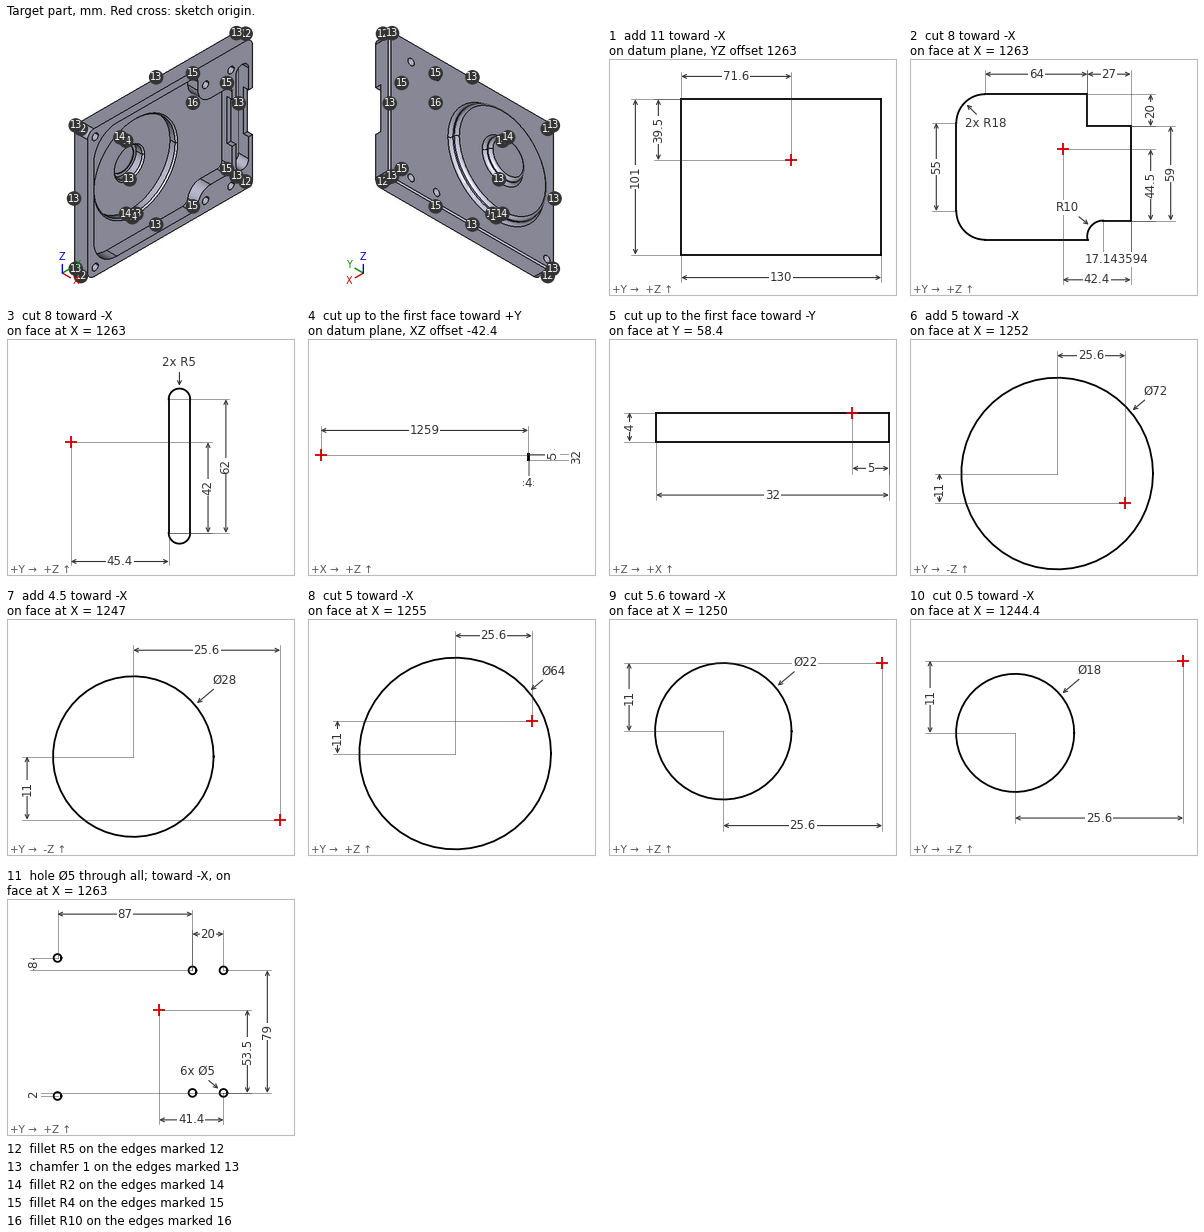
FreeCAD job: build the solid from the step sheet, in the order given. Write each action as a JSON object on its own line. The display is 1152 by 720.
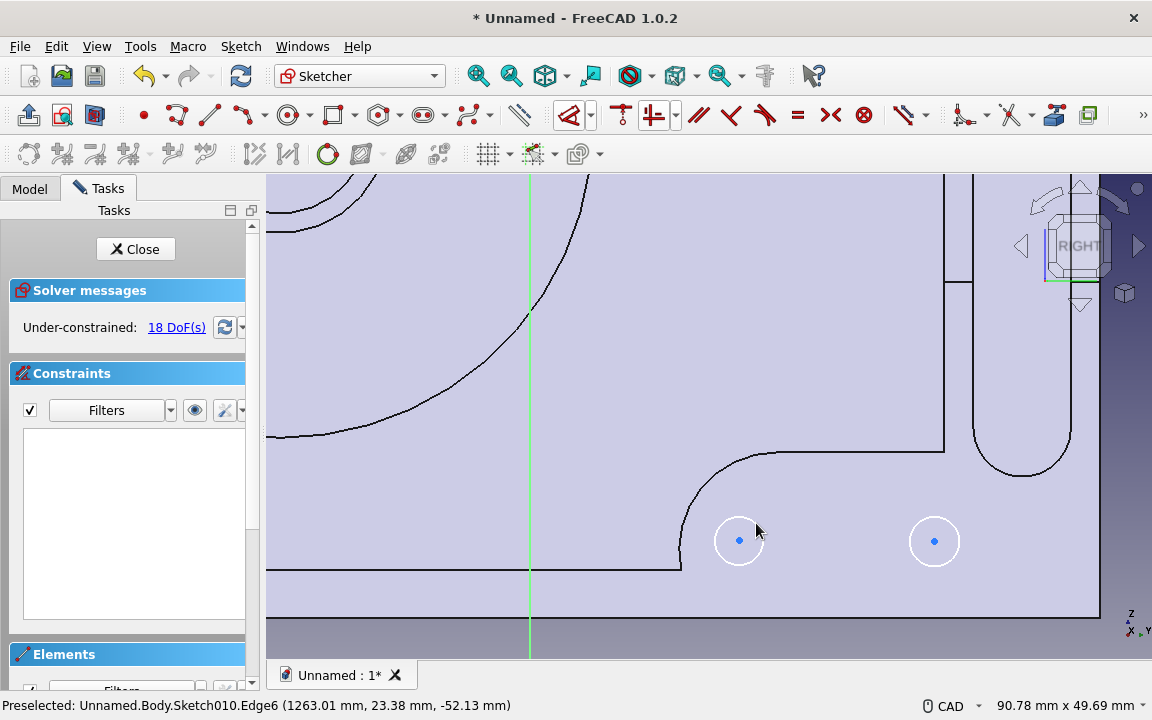
{"action": "left_click", "coordinate": [952, 524]}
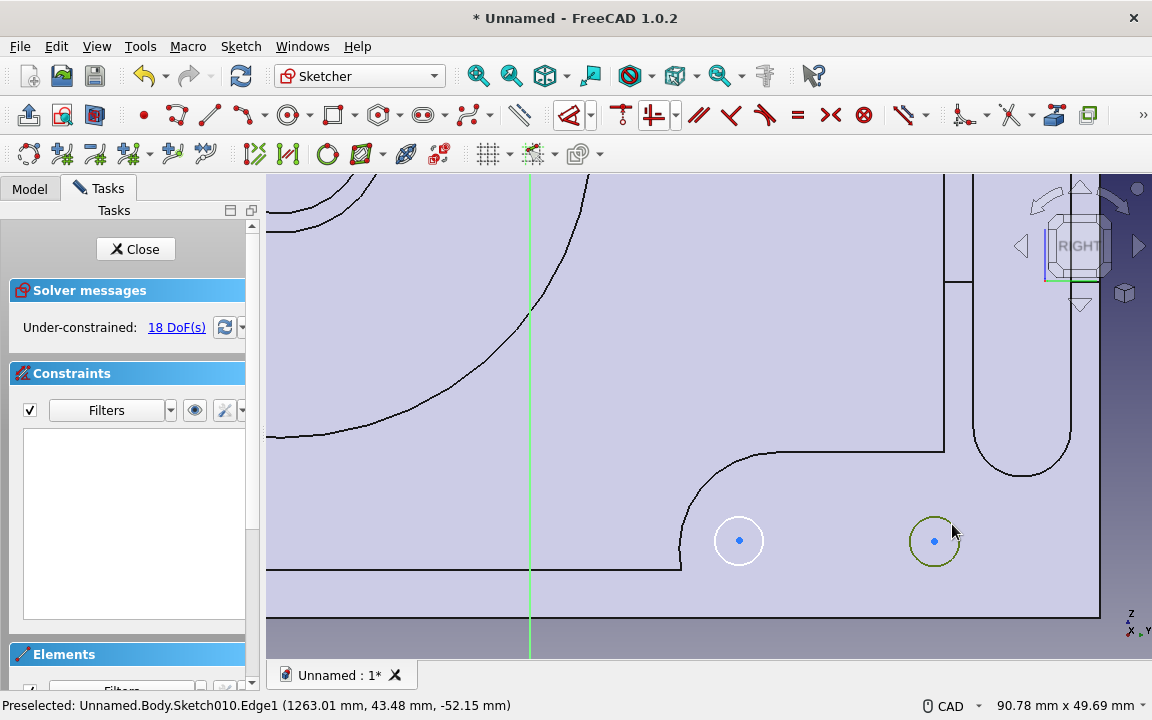
{"action": "scroll", "coordinate": [739, 542], "scroll_direction": "down", "scroll_amount": 6}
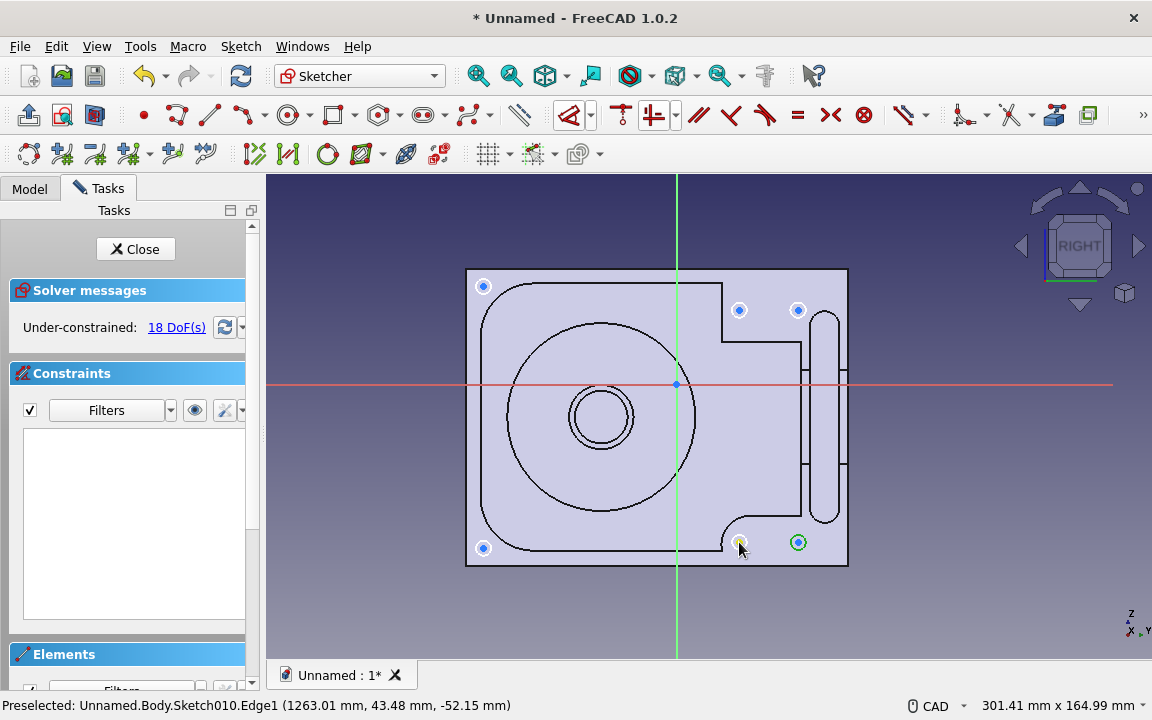
{"action": "scroll", "coordinate": [804, 305], "scroll_direction": "up", "scroll_amount": 3}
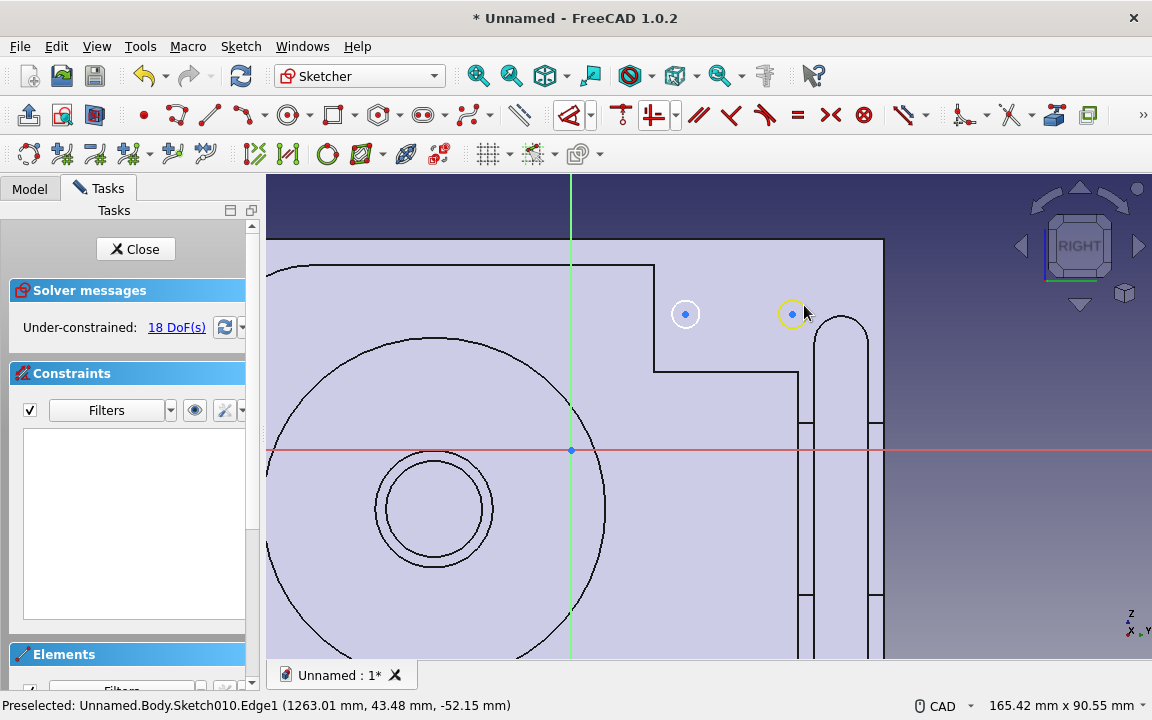
{"action": "left_click", "coordinate": [803, 304]}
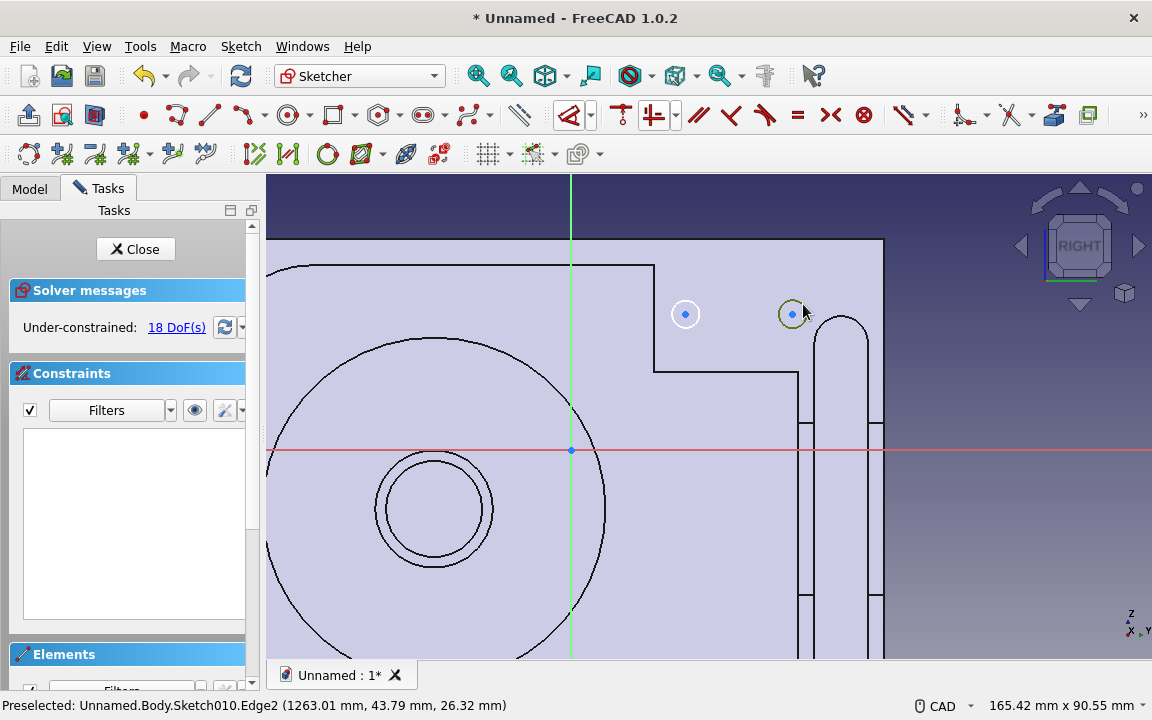
{"action": "left_click", "coordinate": [695, 305]}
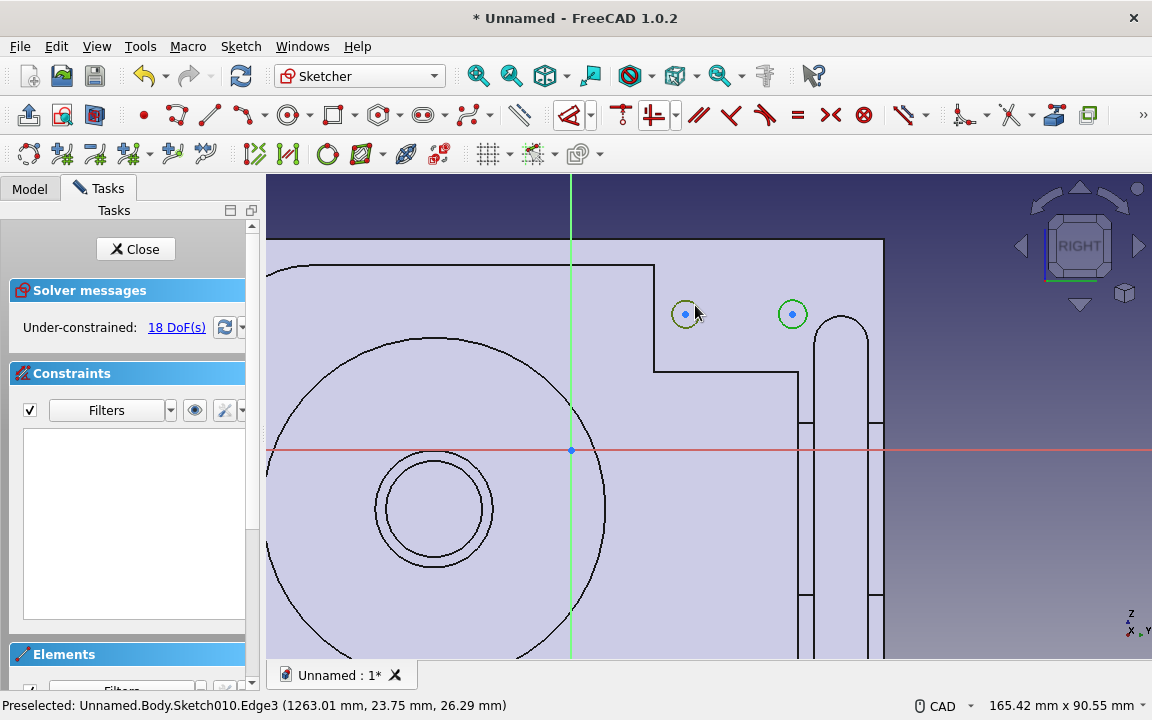
{"action": "scroll", "coordinate": [804, 304], "scroll_direction": "down", "scroll_amount": 3}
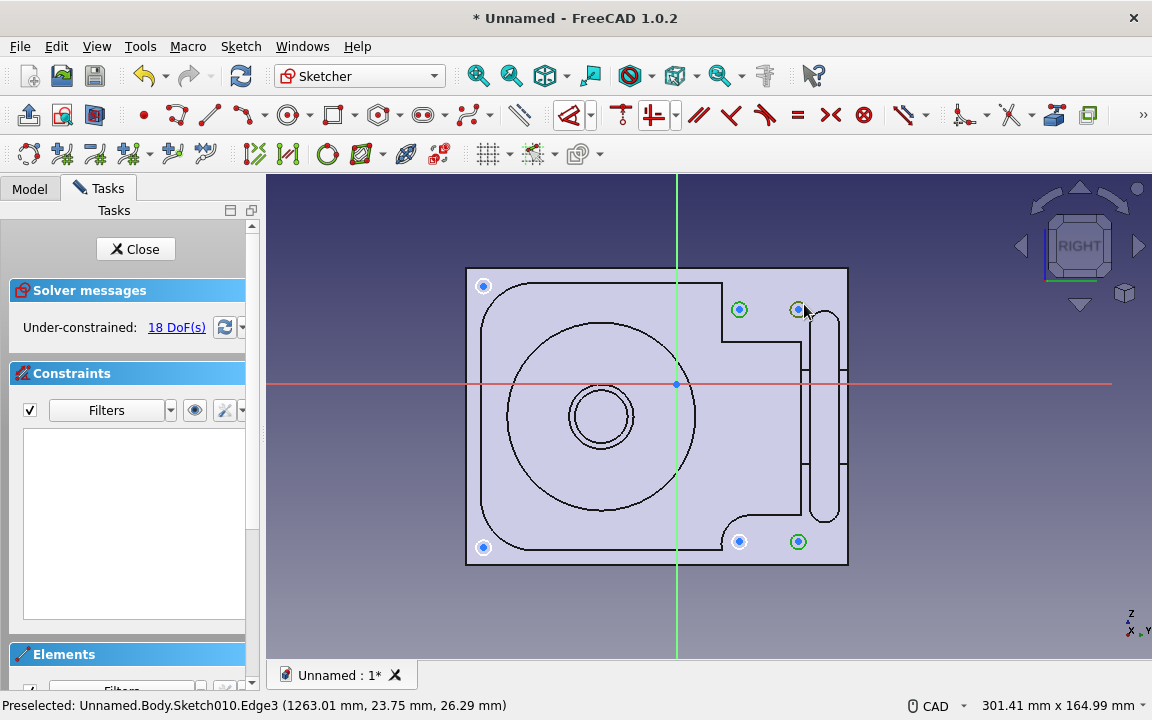
{"action": "scroll", "coordinate": [489, 281], "scroll_direction": "up", "scroll_amount": 4}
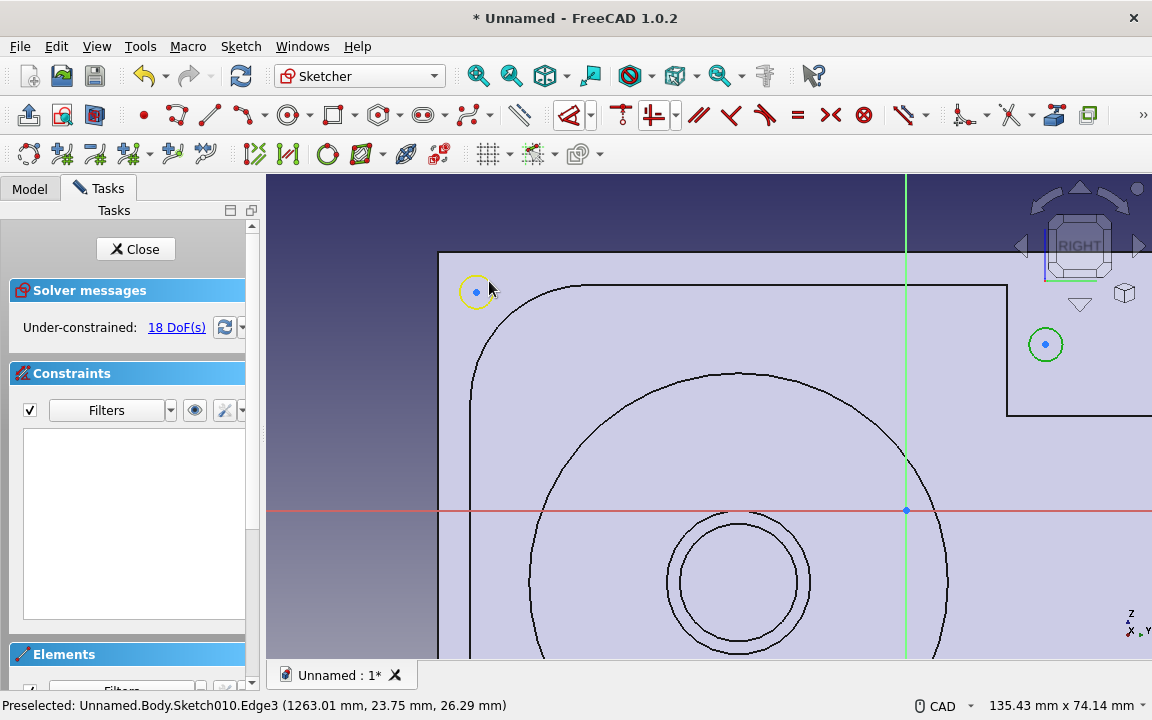
{"action": "left_click", "coordinate": [488, 280]}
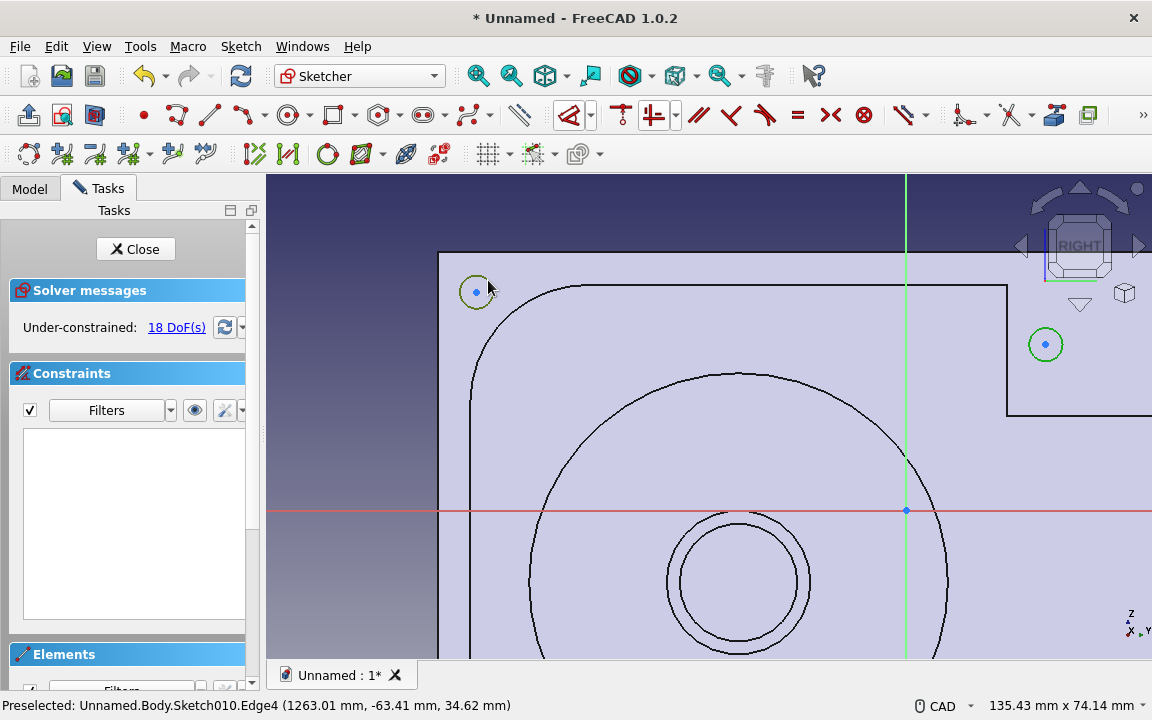
{"action": "scroll", "coordinate": [488, 281], "scroll_direction": "down", "scroll_amount": 4}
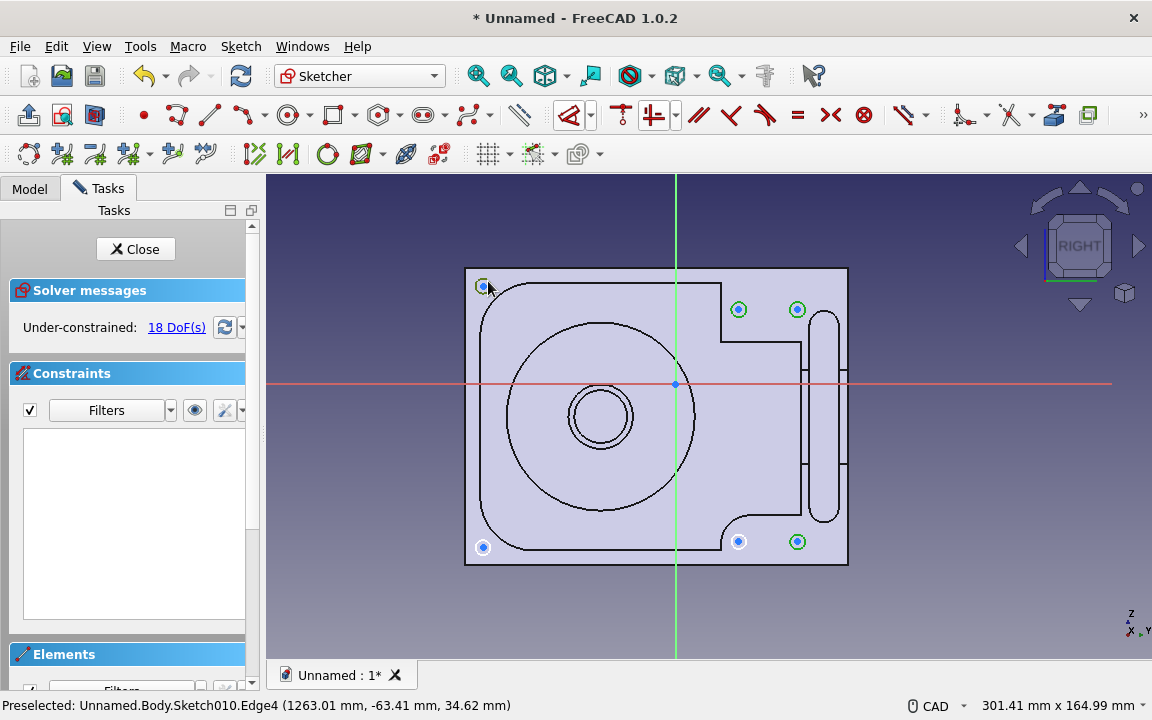
{"action": "scroll", "coordinate": [488, 542], "scroll_direction": "up", "scroll_amount": 4}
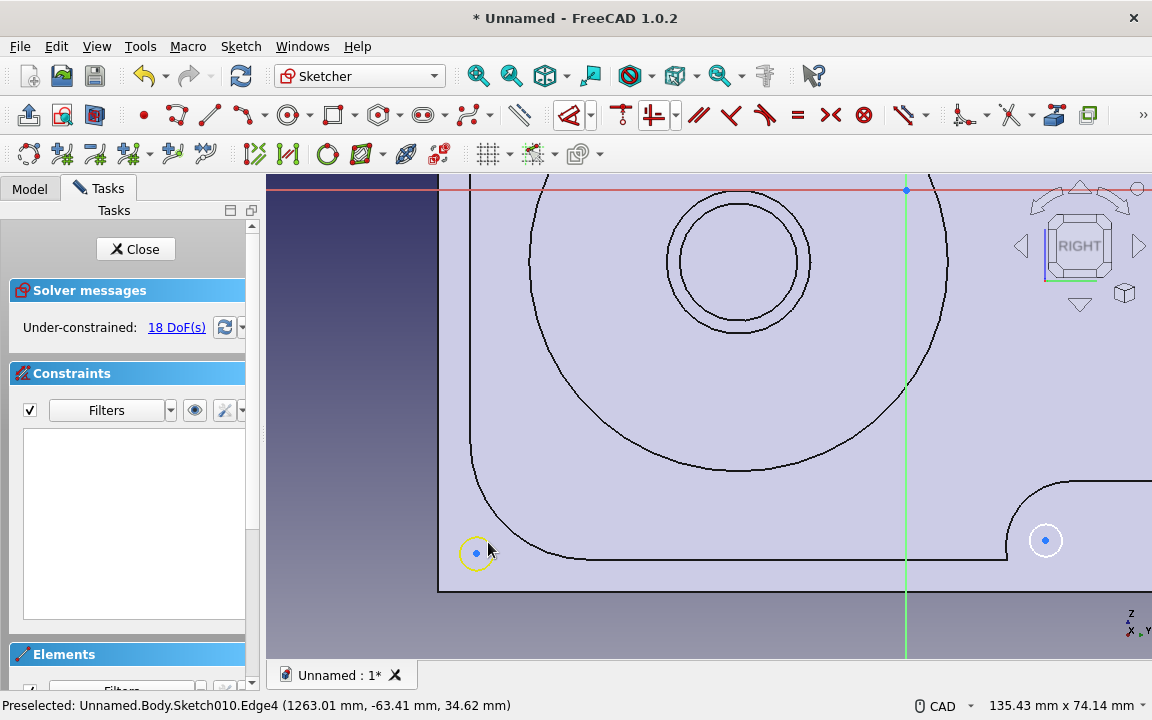
{"action": "left_click", "coordinate": [488, 542]}